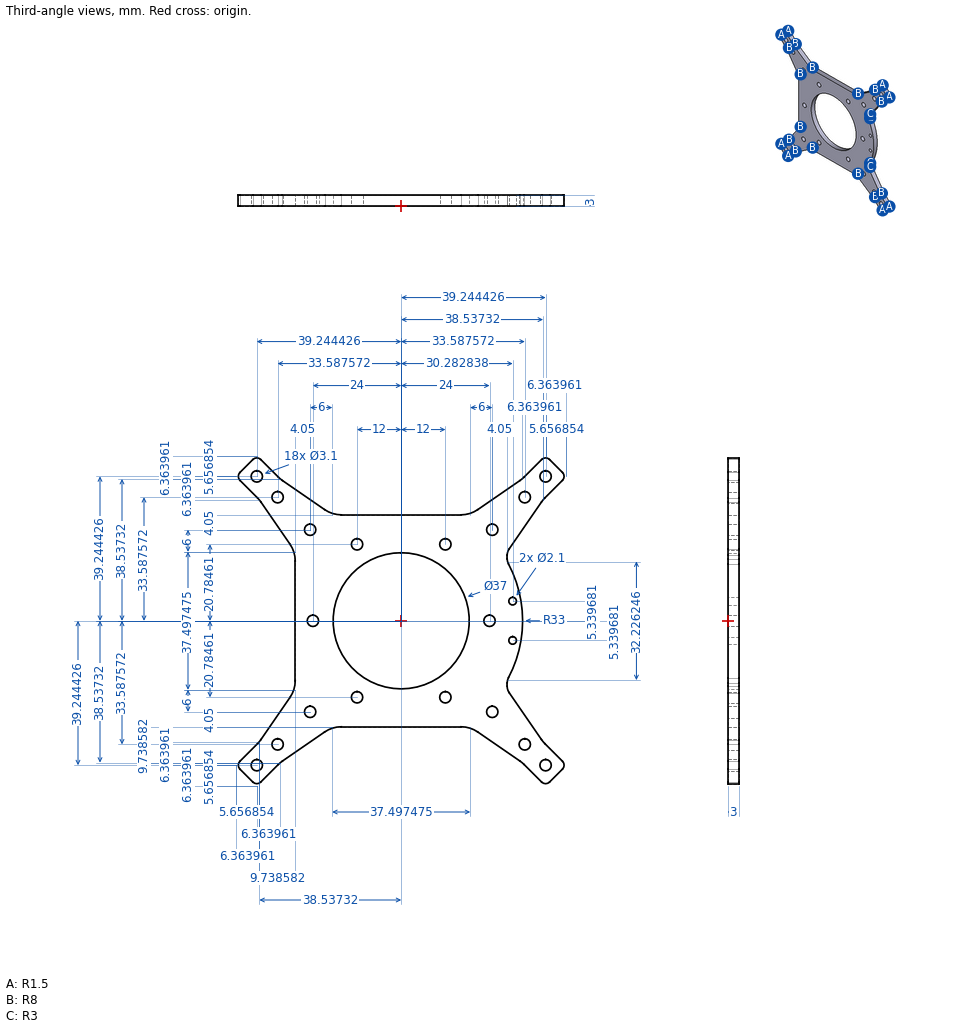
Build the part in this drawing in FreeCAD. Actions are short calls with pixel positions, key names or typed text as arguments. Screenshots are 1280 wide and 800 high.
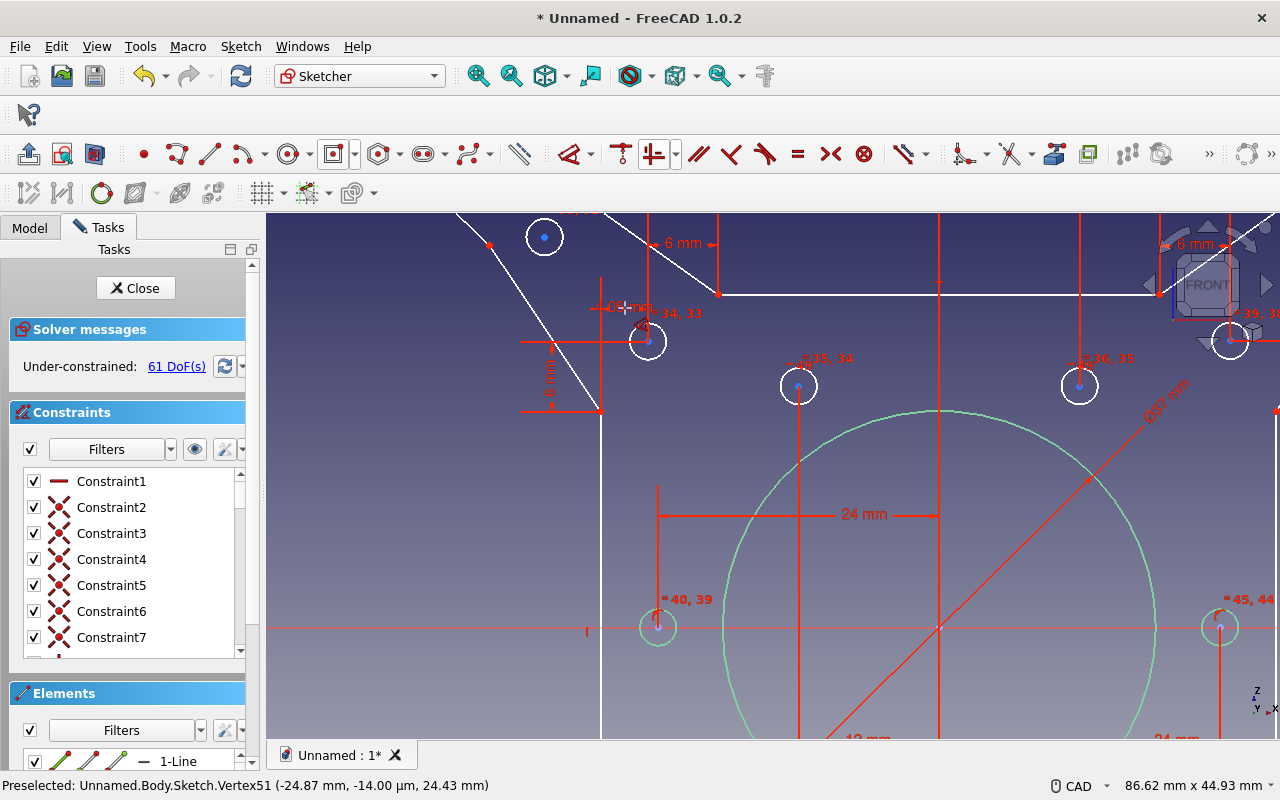
click(718, 295)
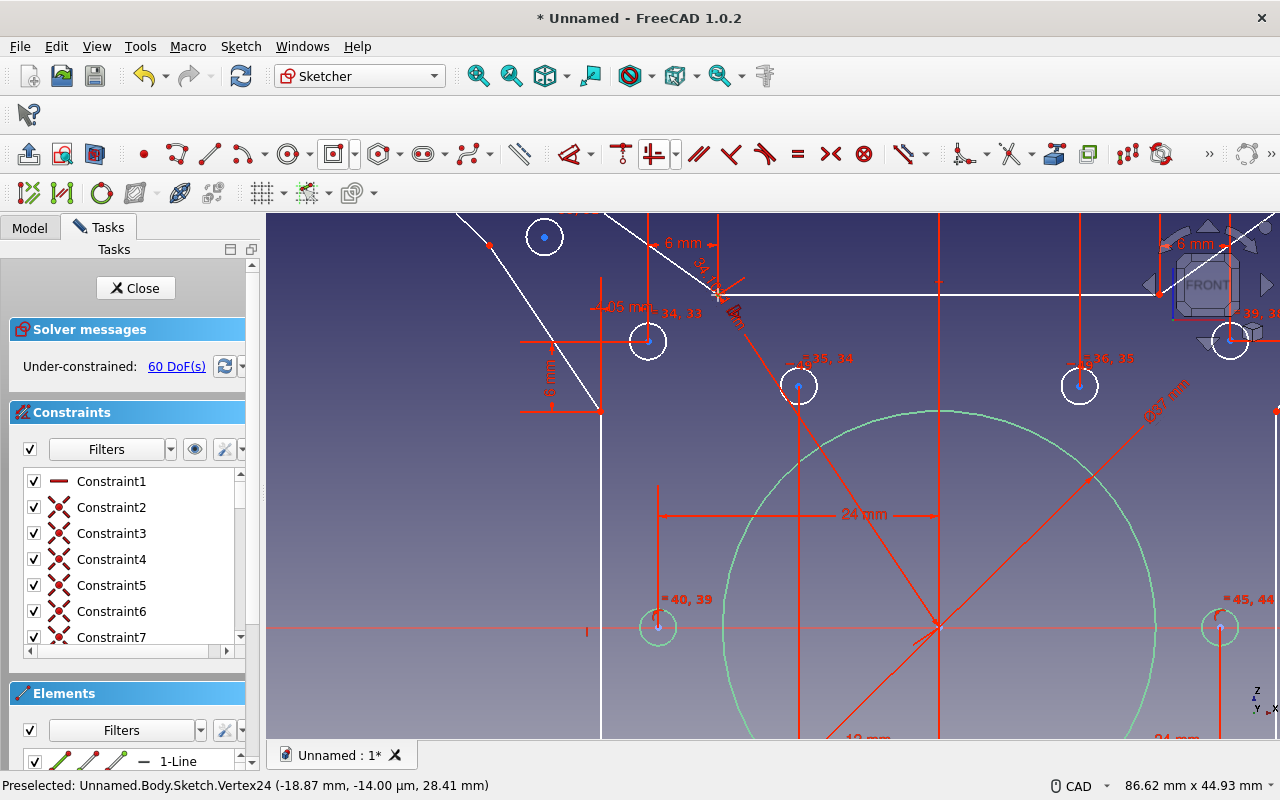
click(648, 342)
click(614, 329)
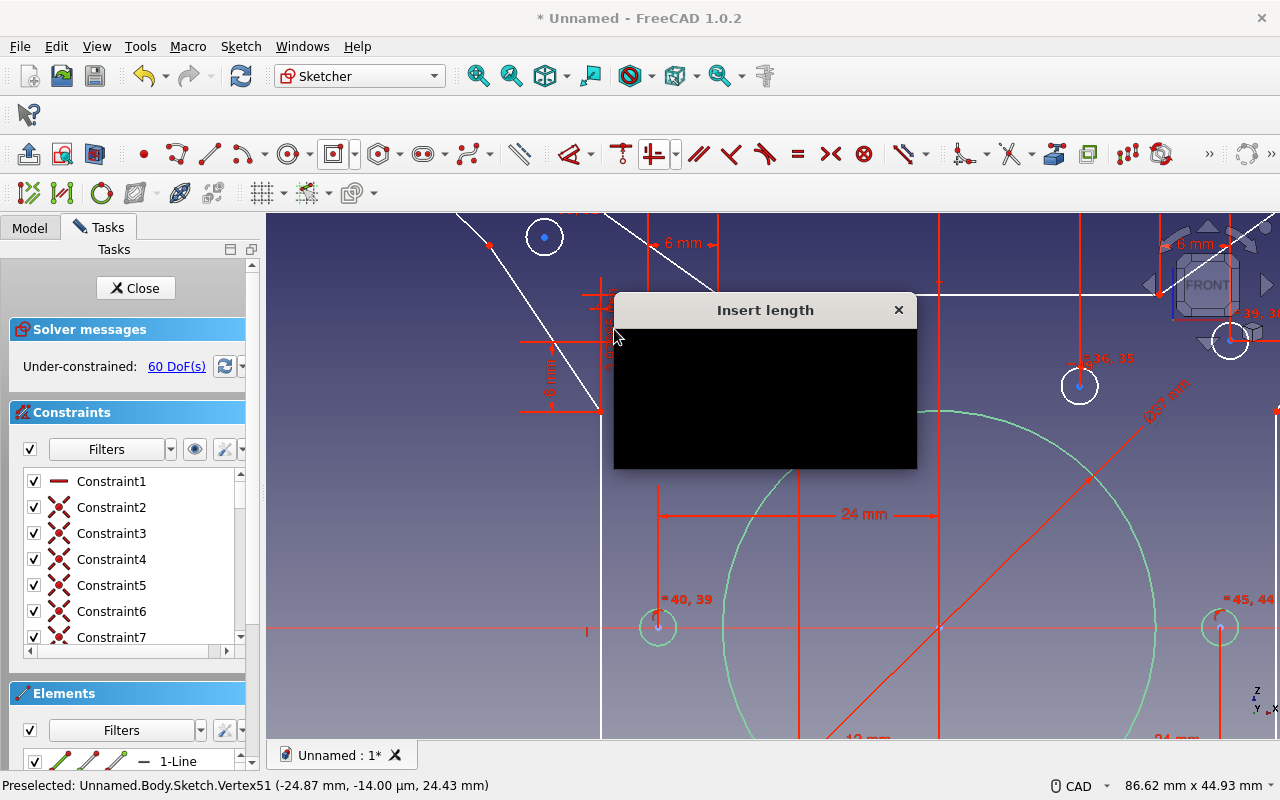
text(4.05)
key(Return)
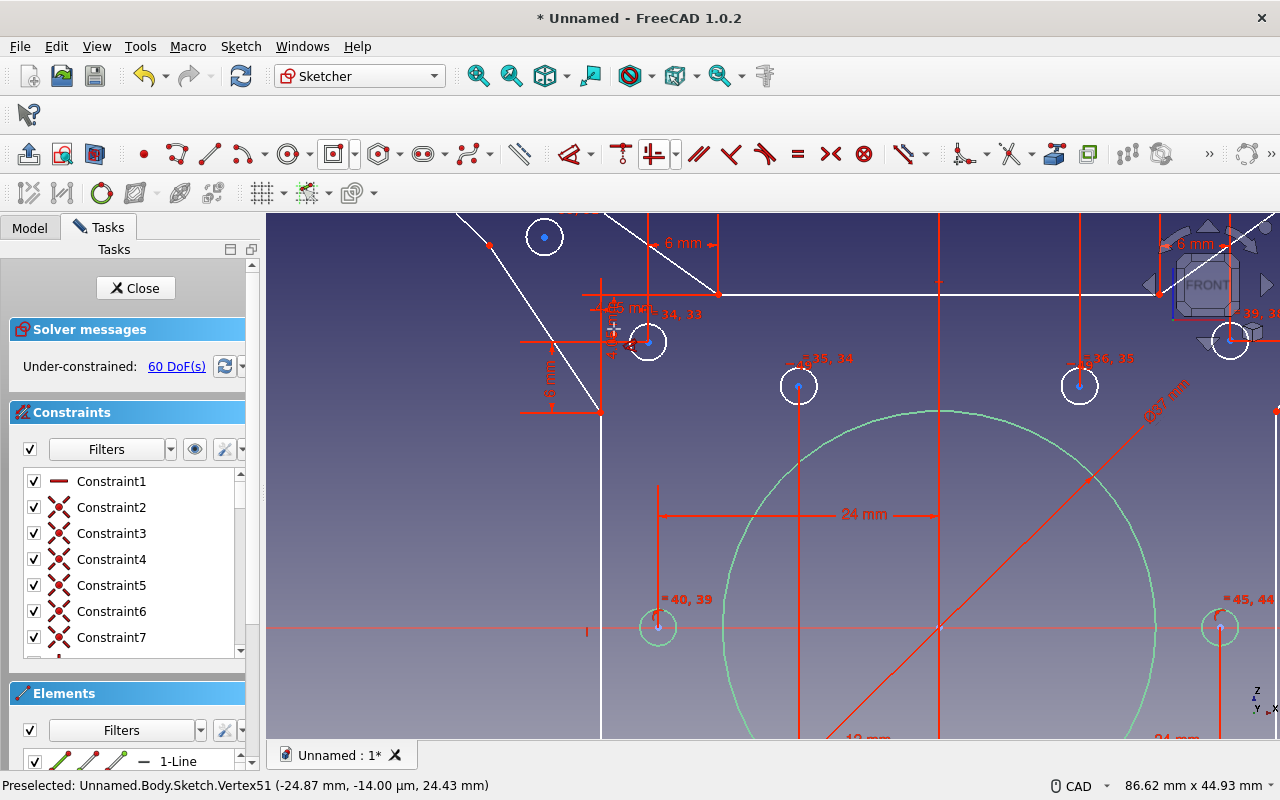
scroll(603, 411, down, 6)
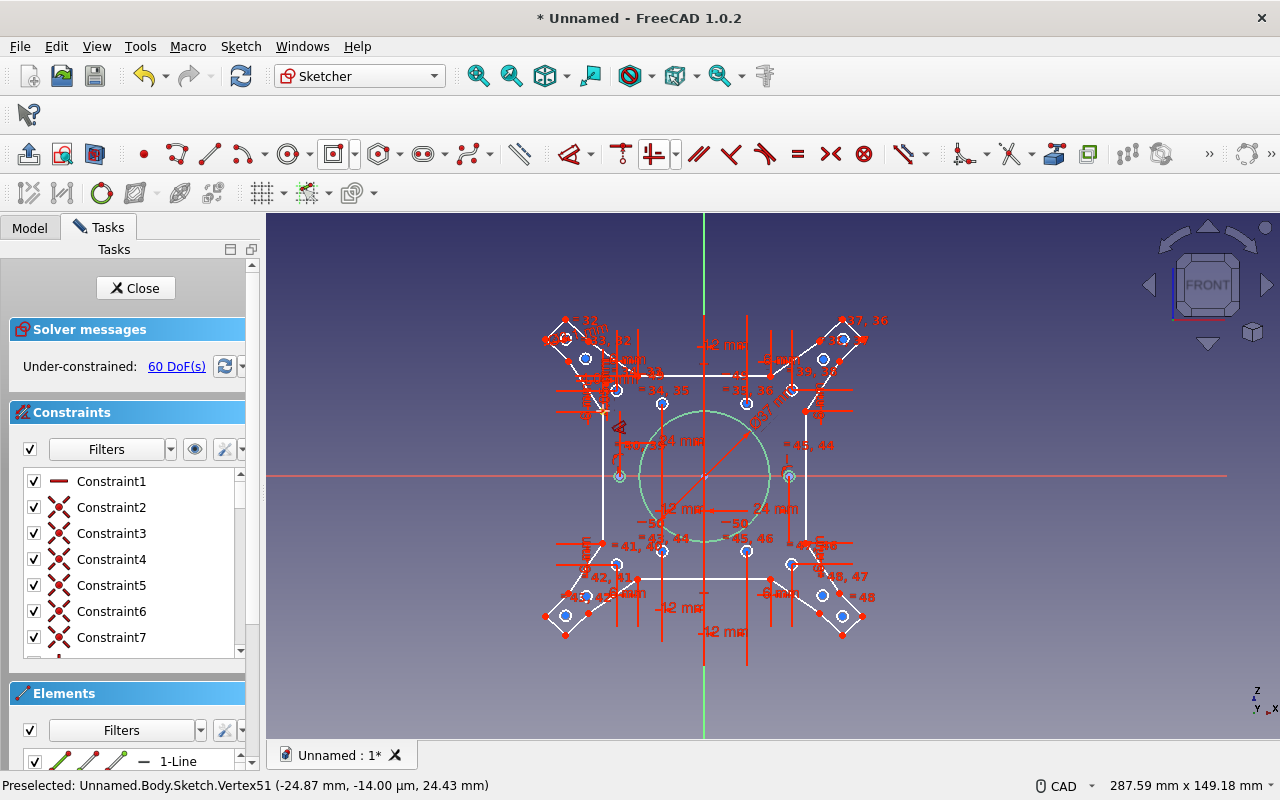
scroll(806, 411, up, 6)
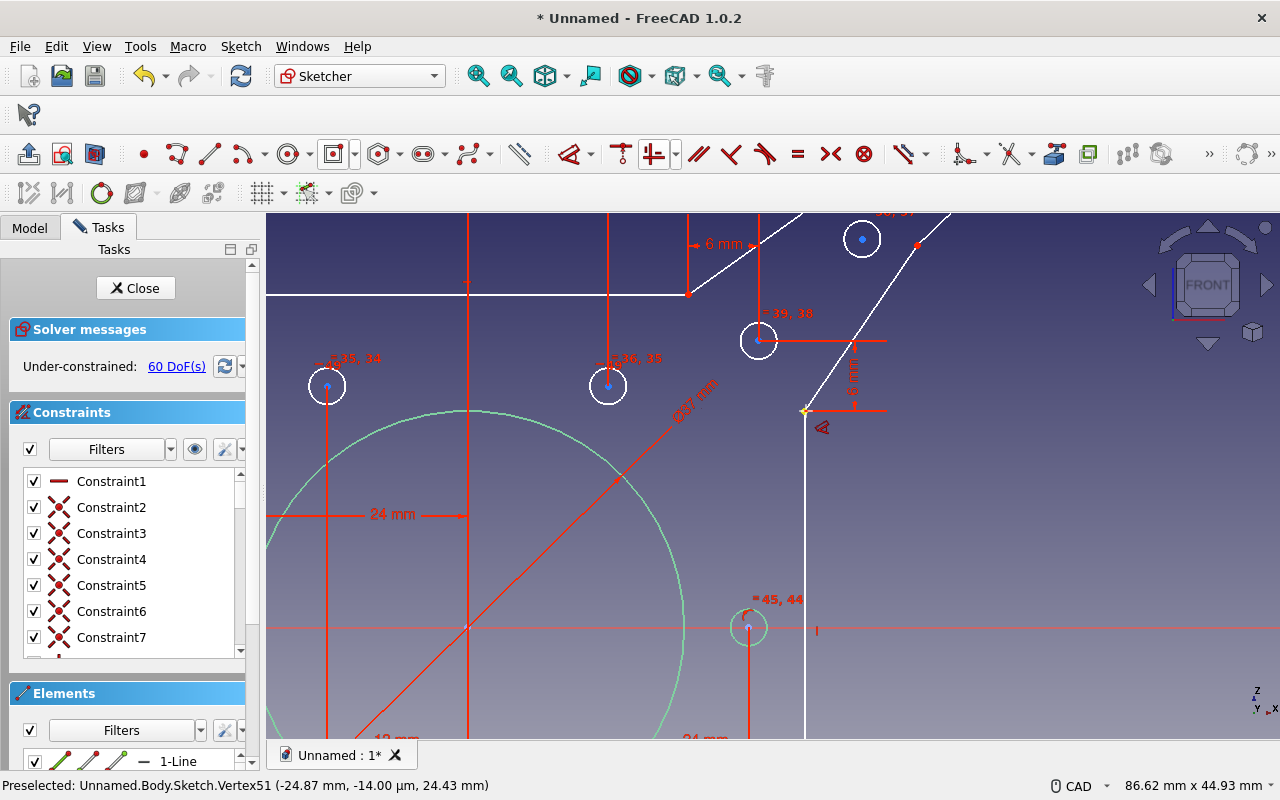
click(805, 411)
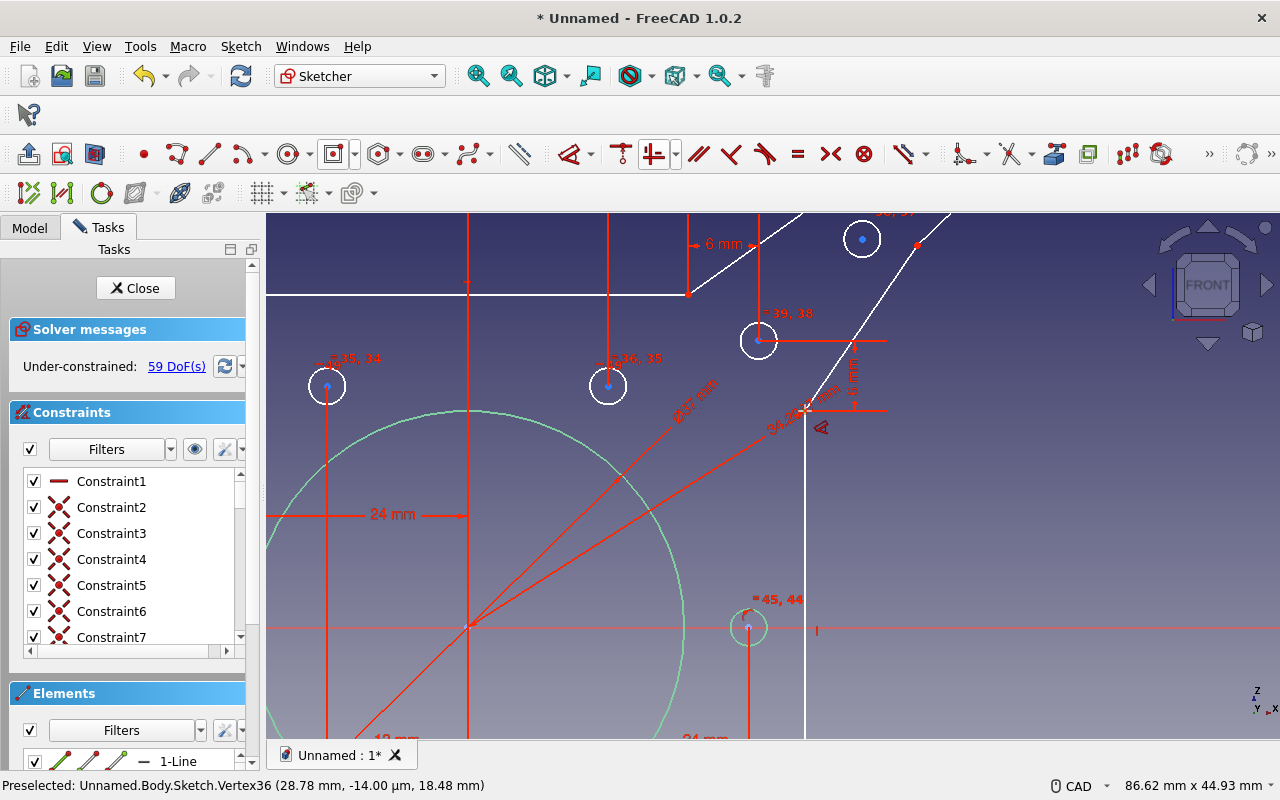
click(759, 341)
click(782, 307)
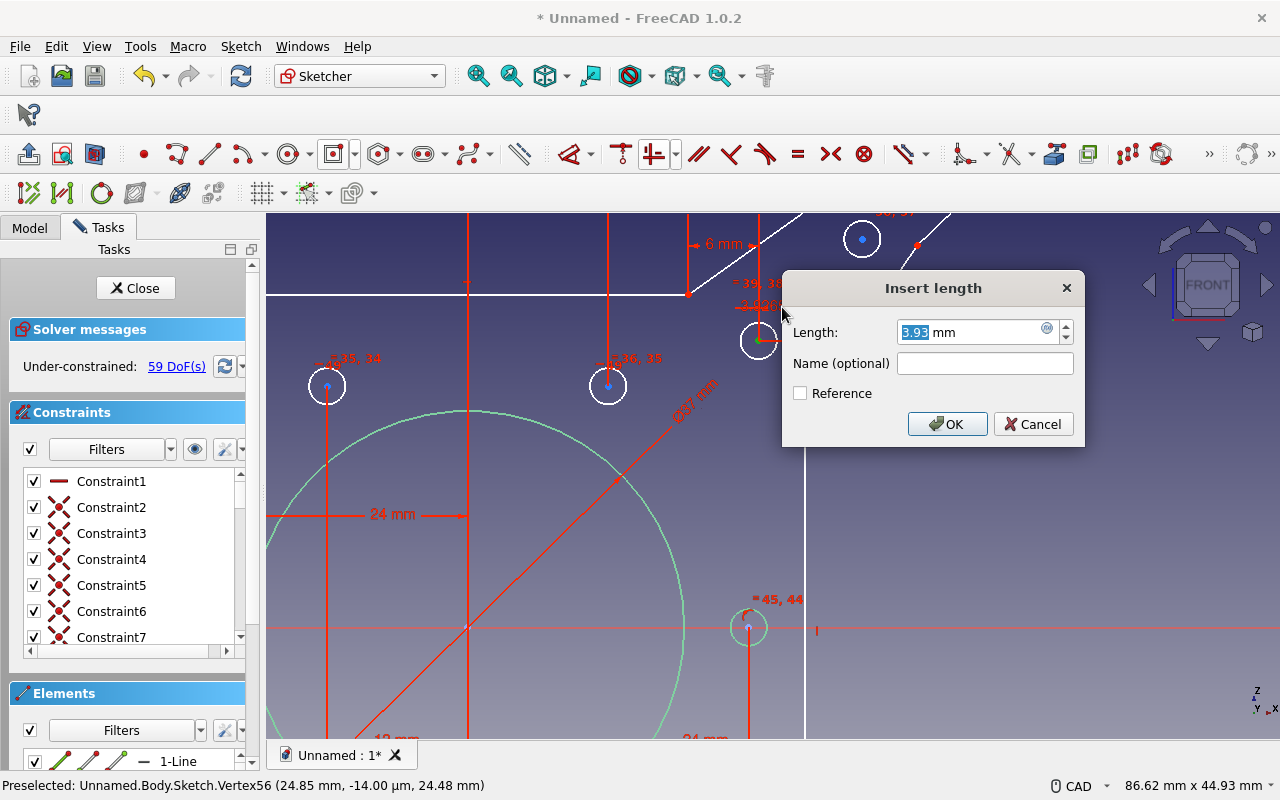
text(4.05)
key(Return)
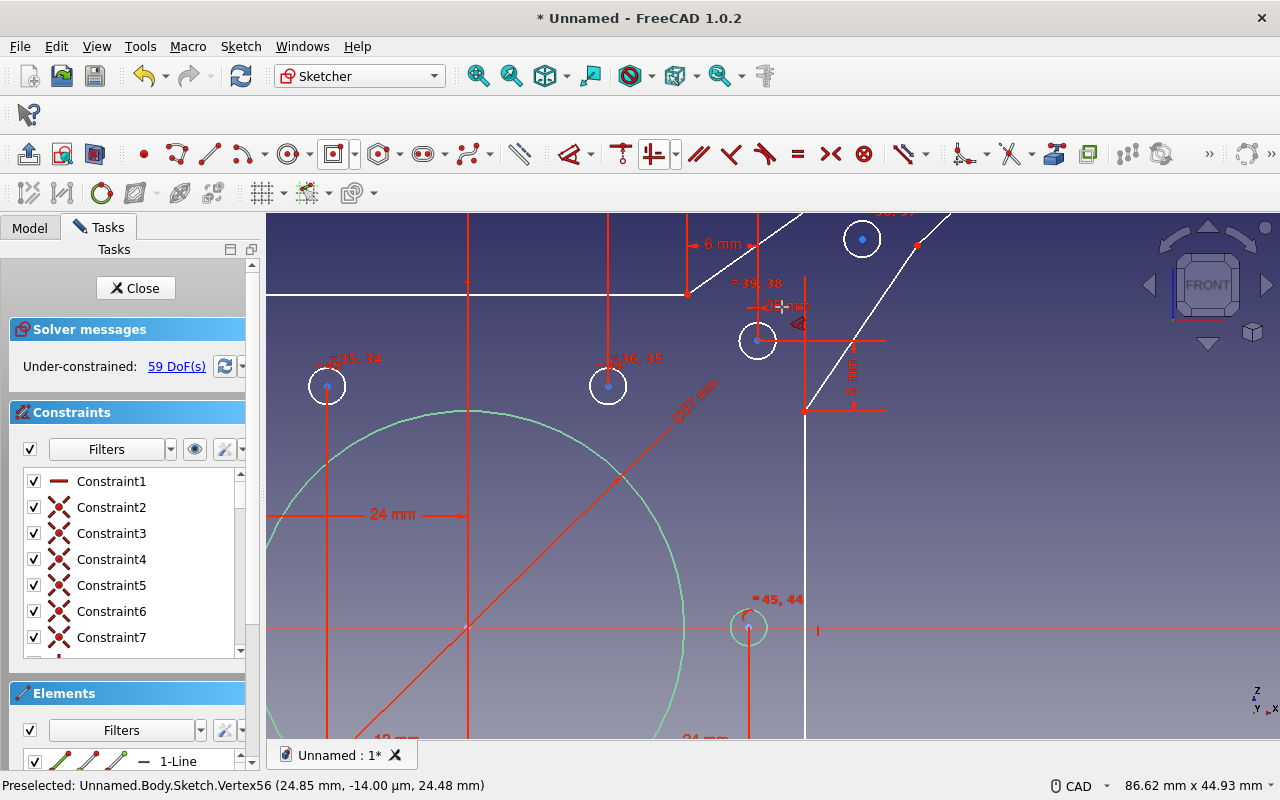
click(687, 295)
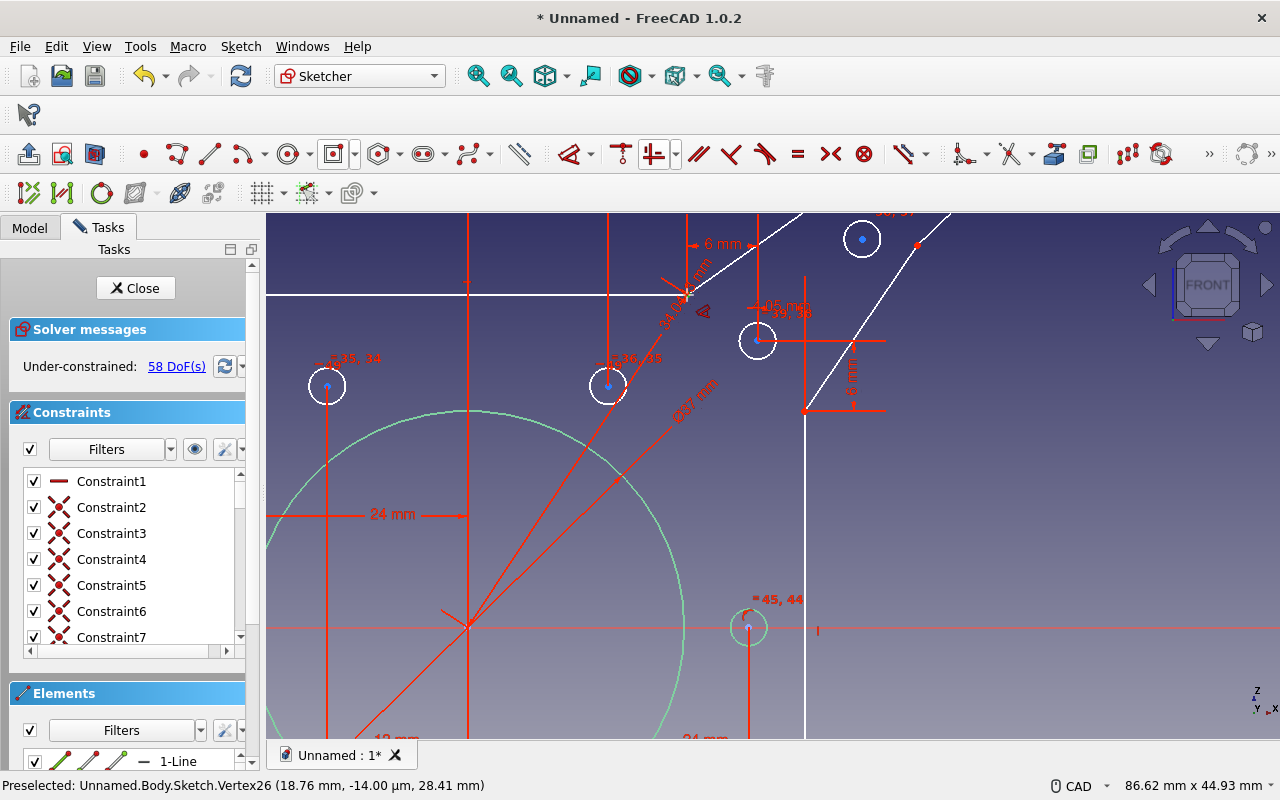
click(758, 341)
click(792, 329)